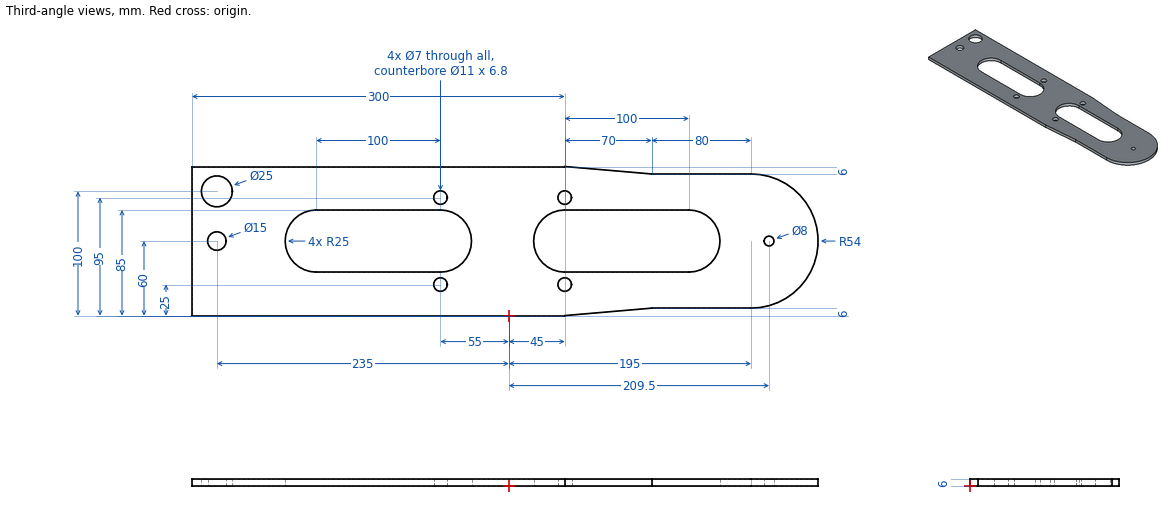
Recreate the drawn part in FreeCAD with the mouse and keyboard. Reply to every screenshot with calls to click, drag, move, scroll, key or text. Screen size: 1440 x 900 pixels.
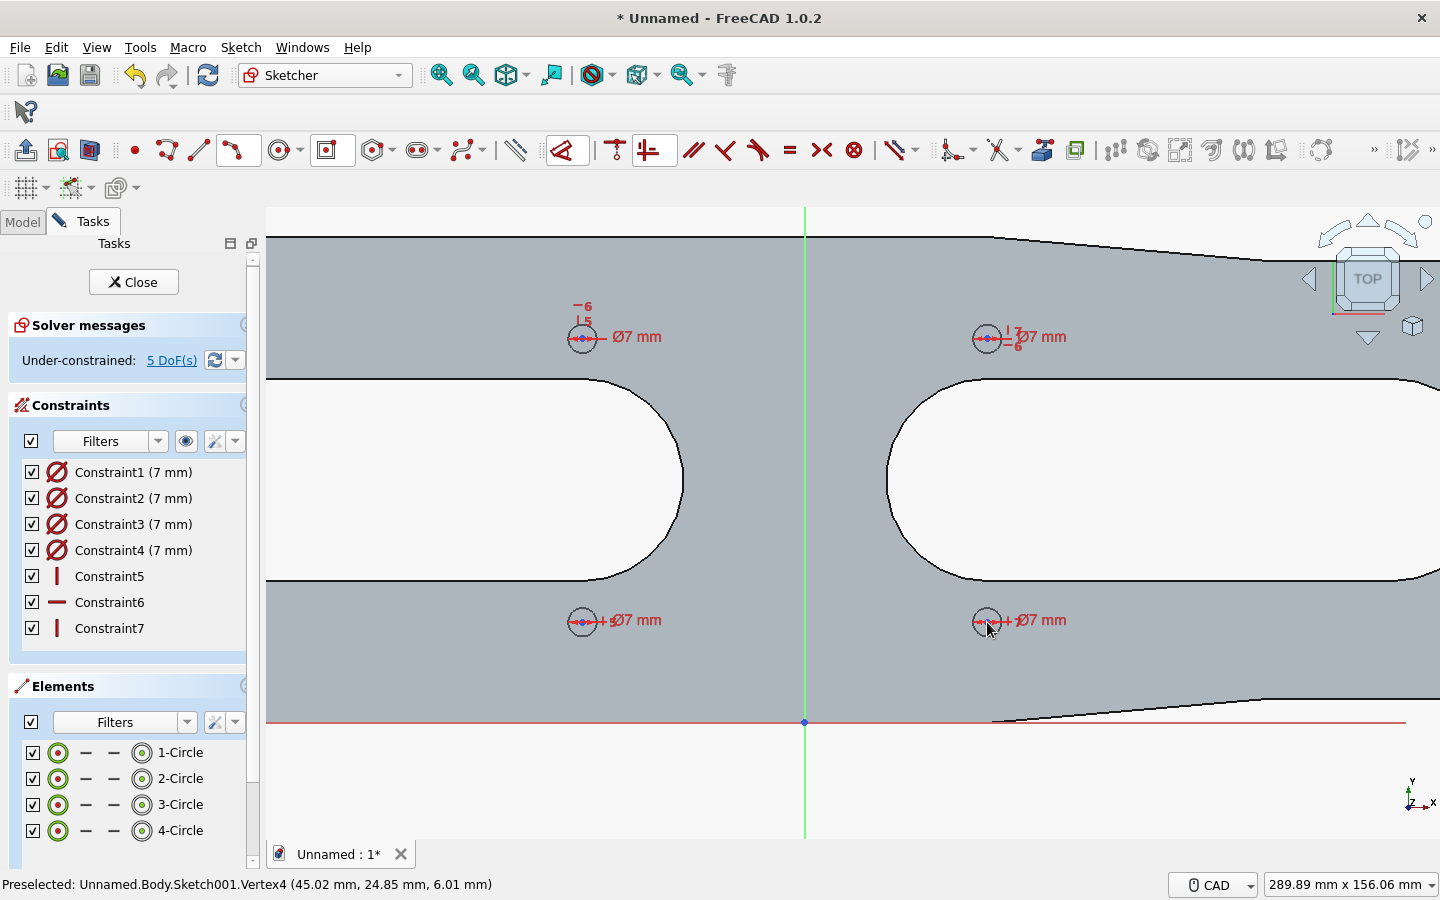
click(582, 622)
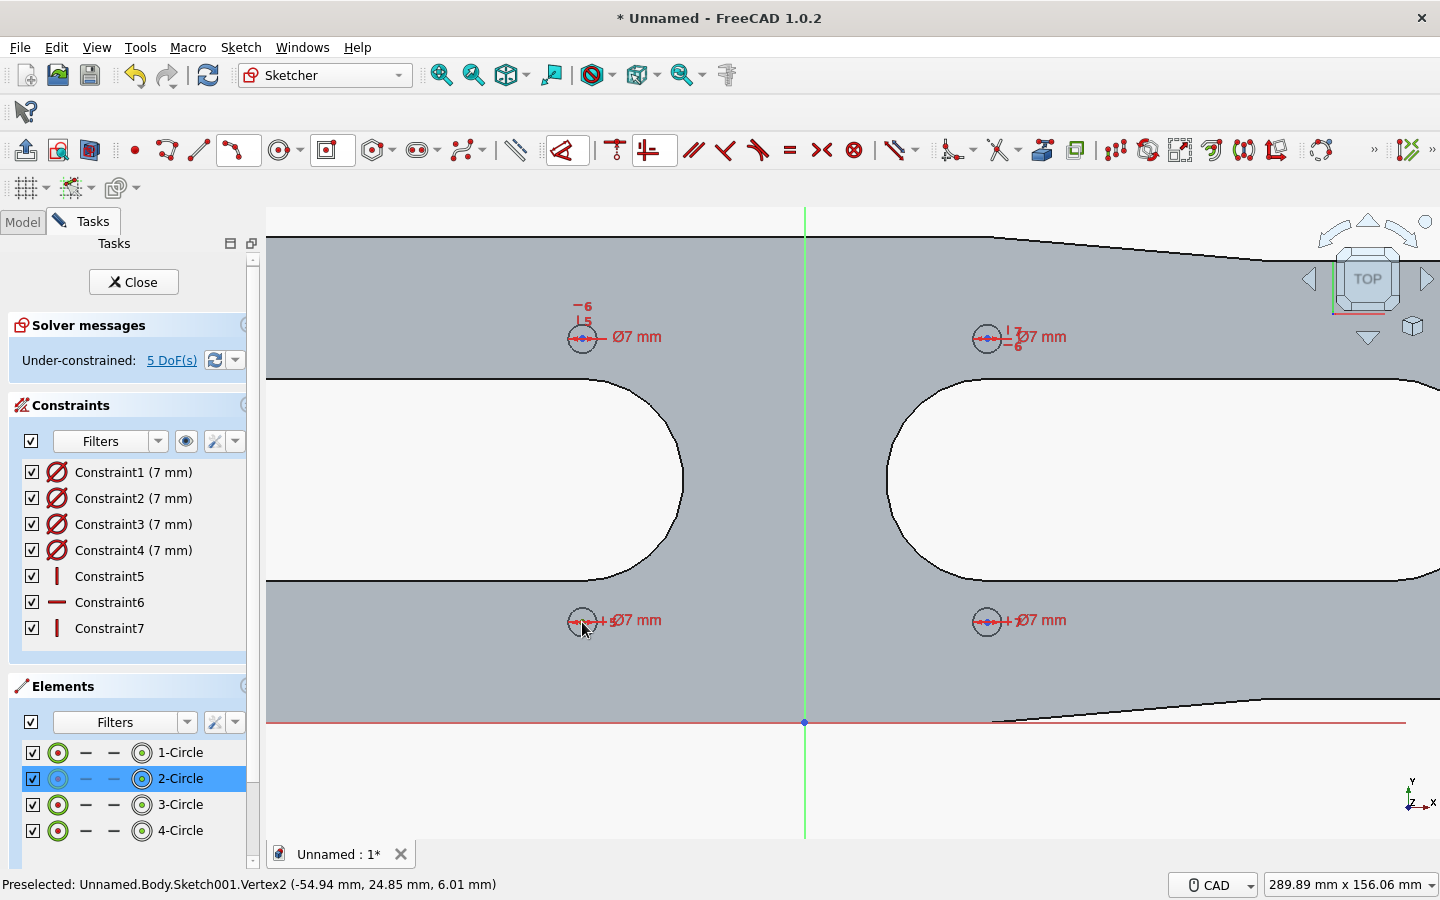
click(987, 622)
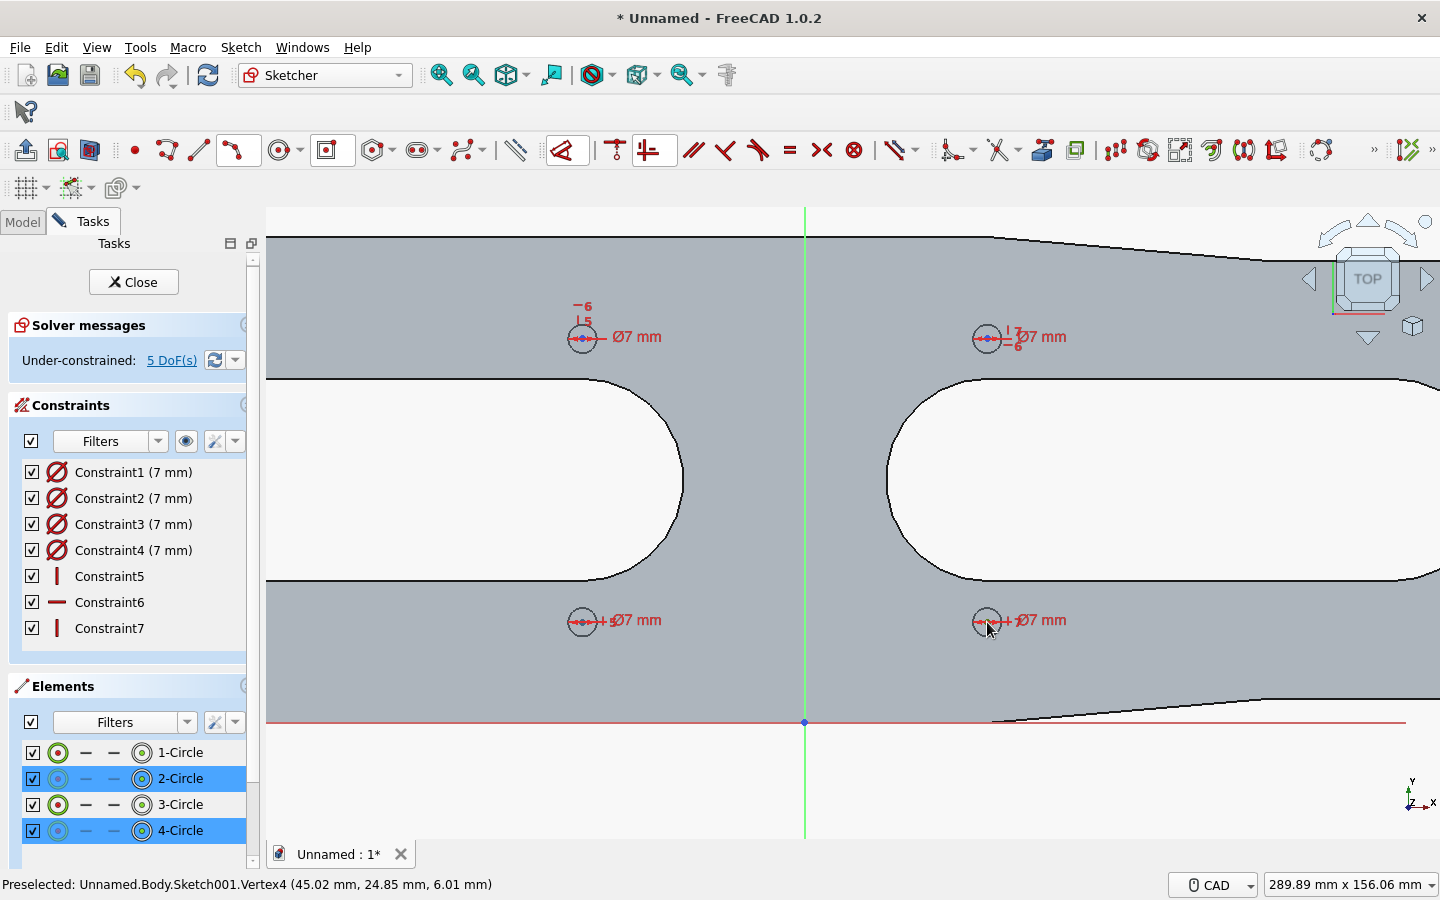
key(h)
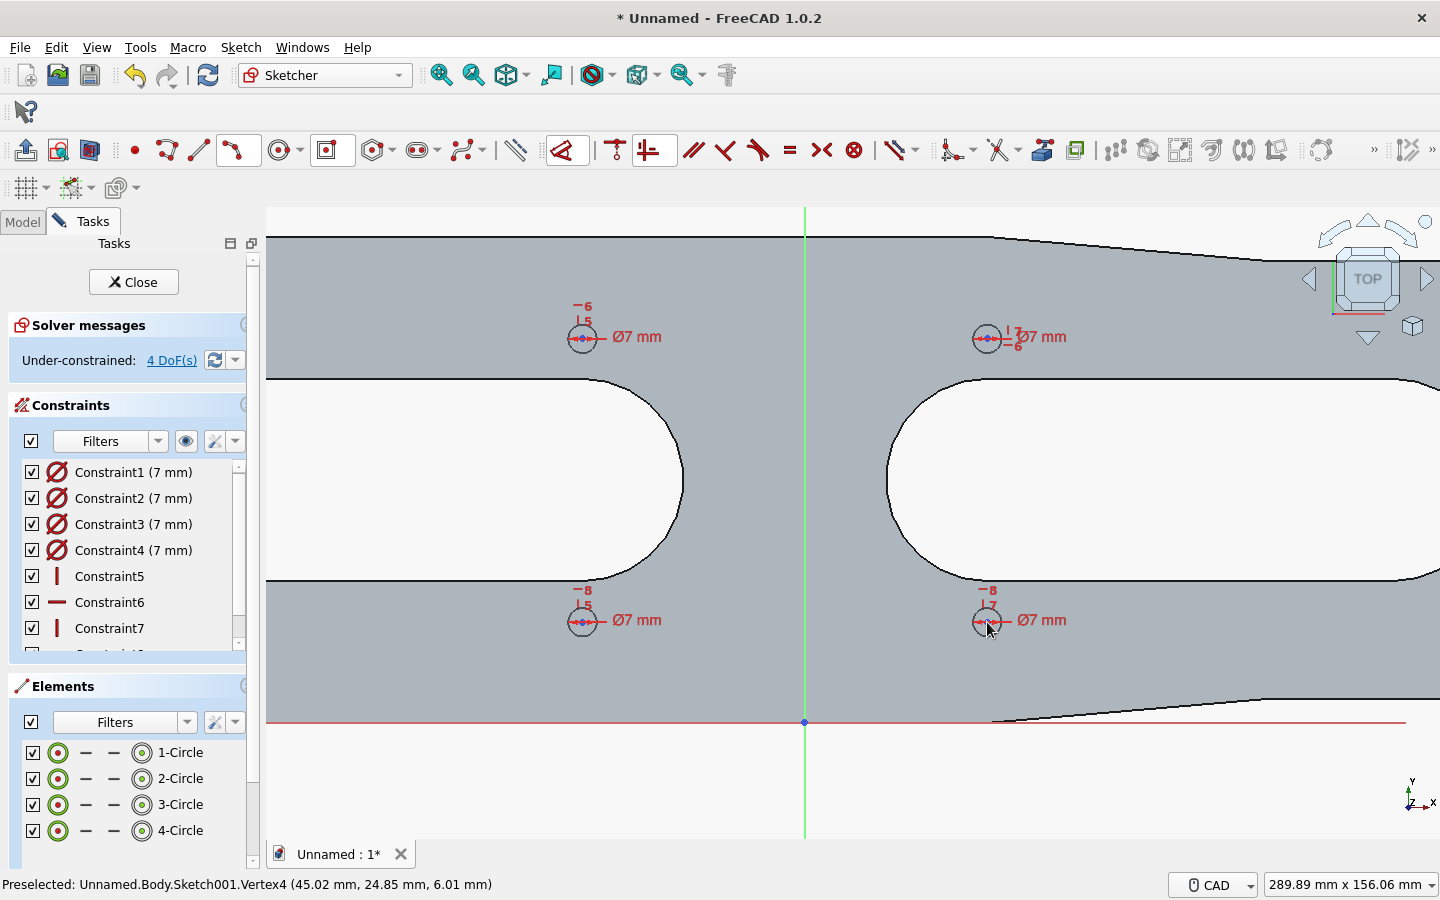
click(582, 339)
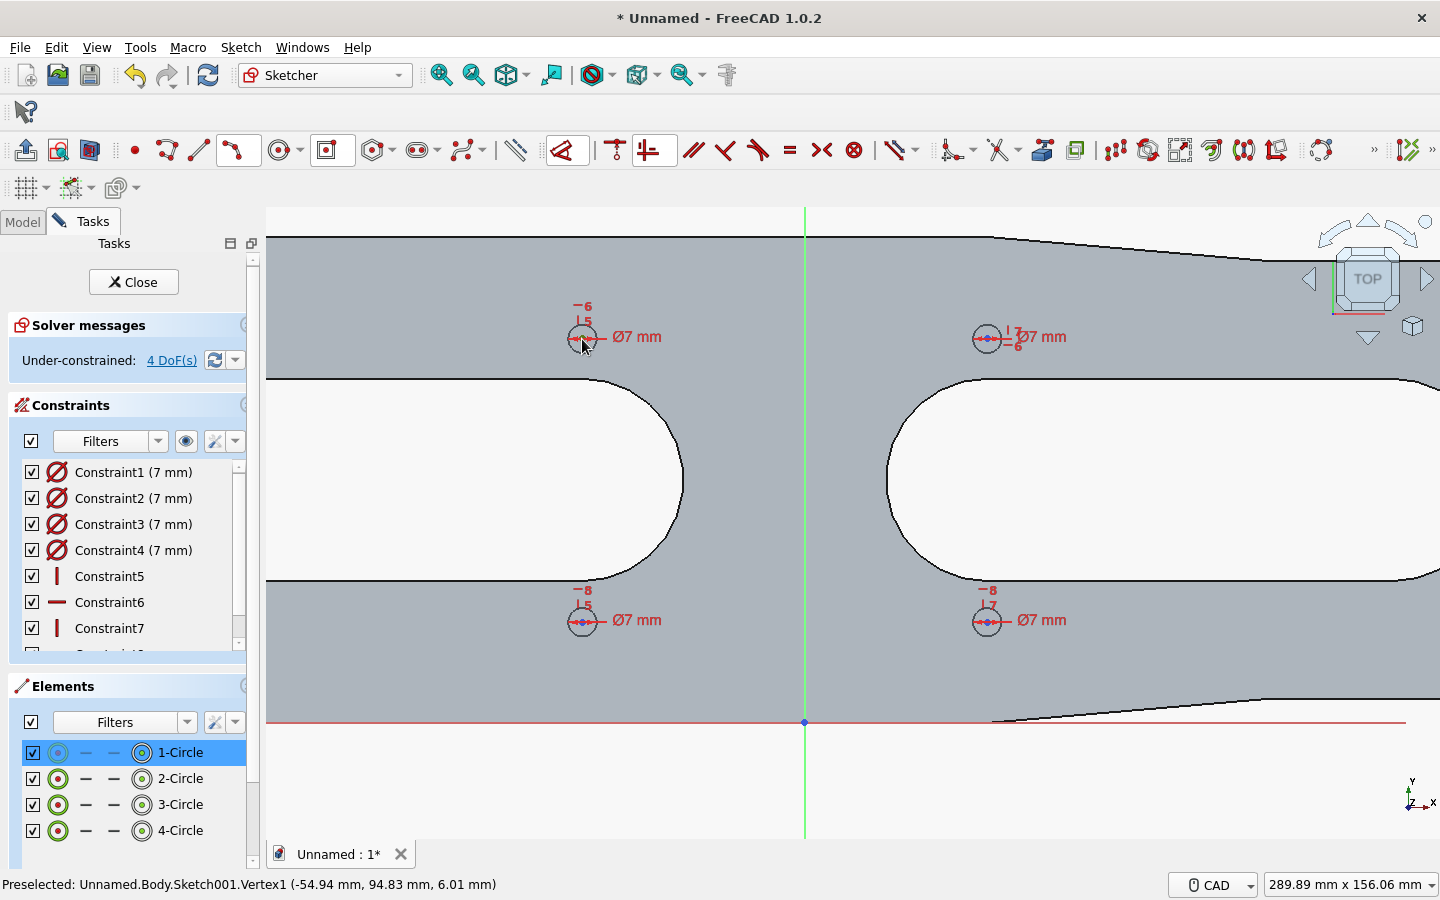
click(584, 150)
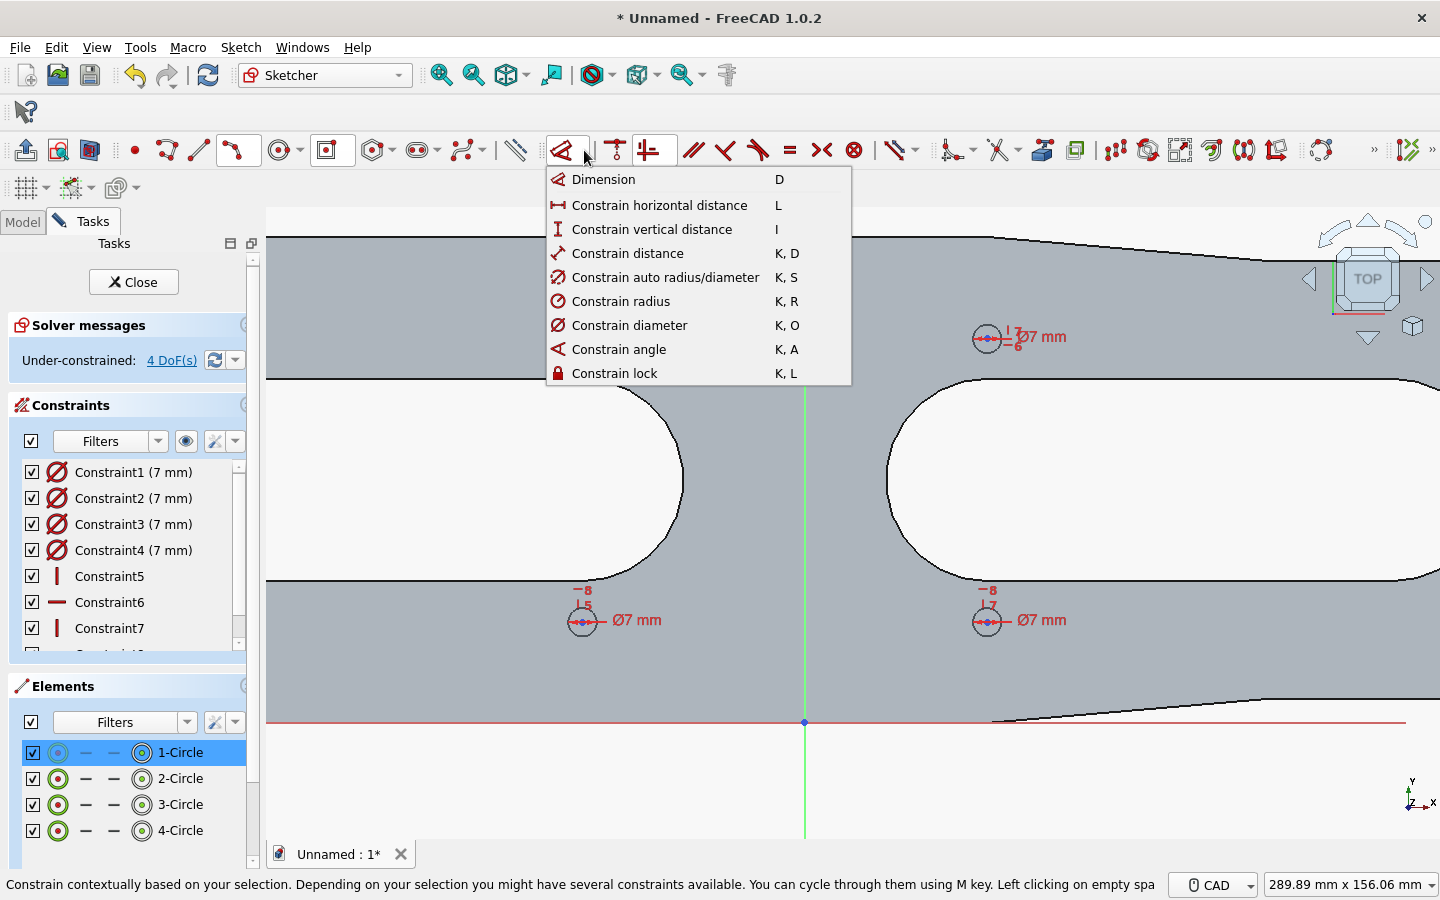
click(699, 205)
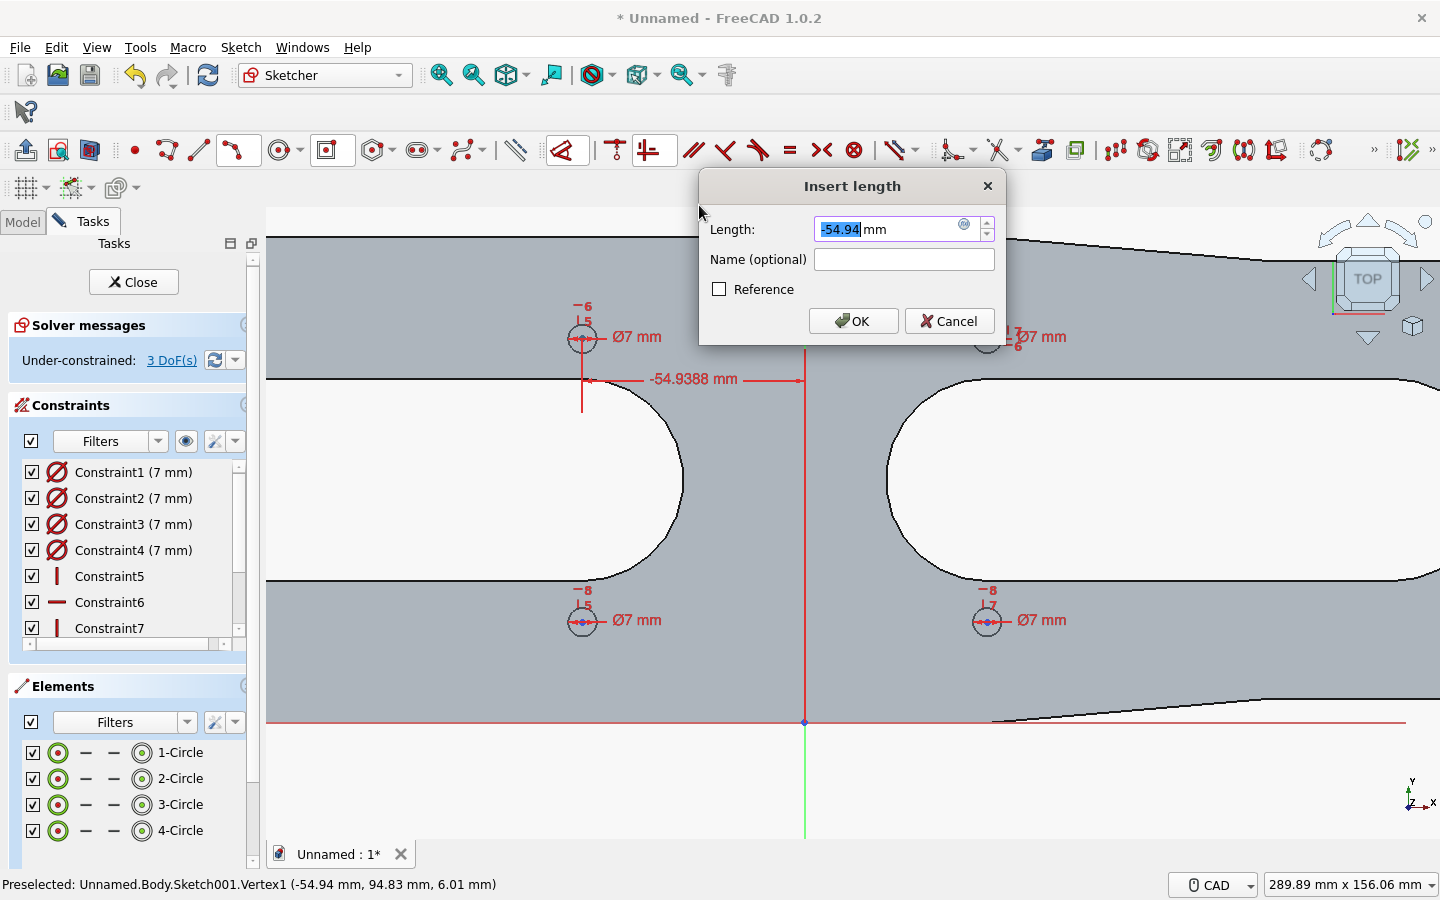
text(-55)
key(Return)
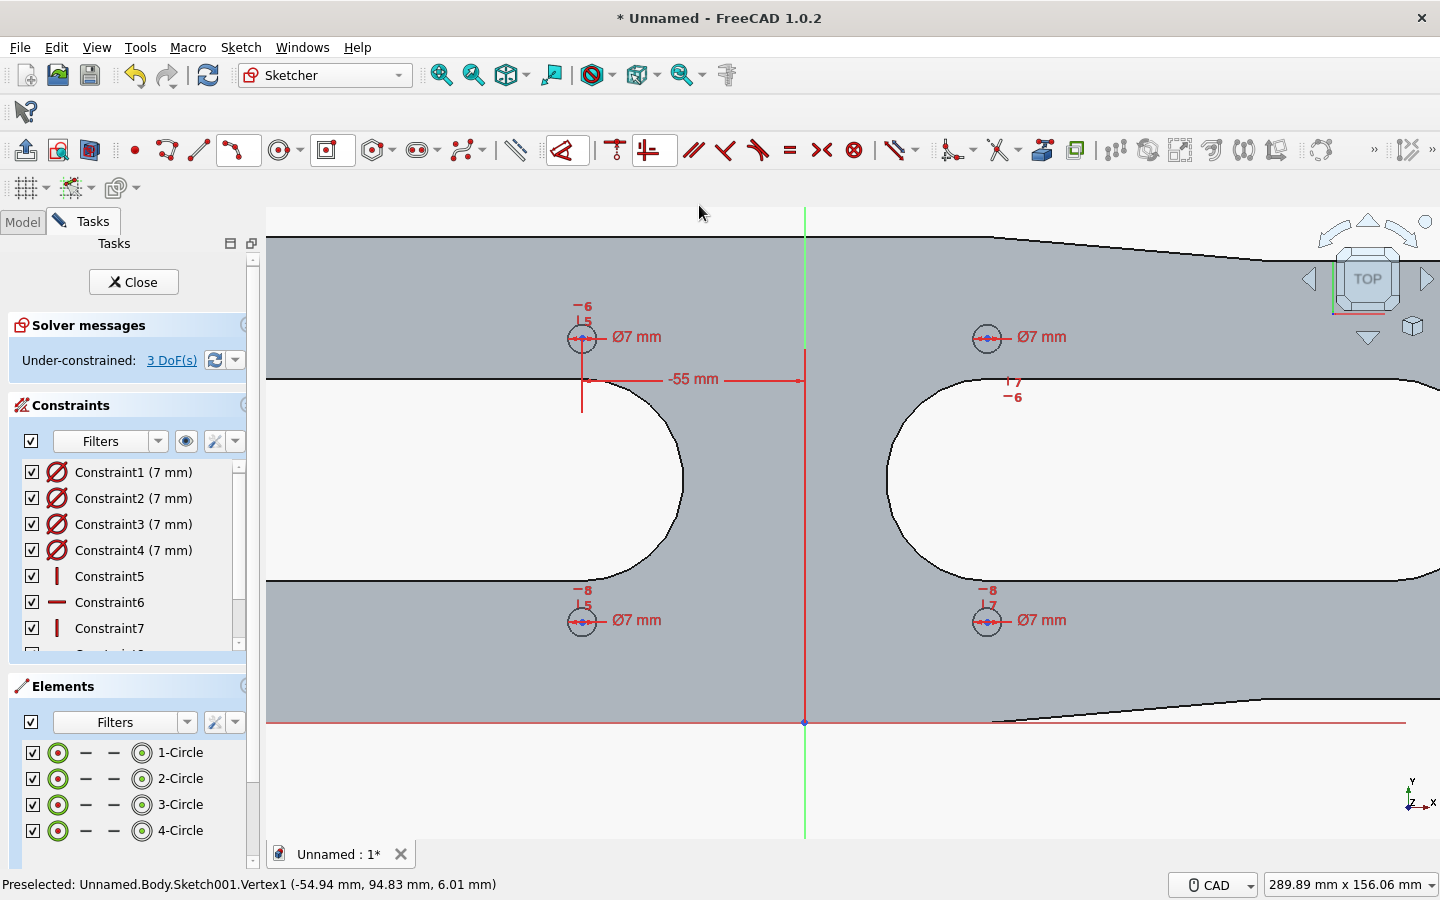
click(582, 339)